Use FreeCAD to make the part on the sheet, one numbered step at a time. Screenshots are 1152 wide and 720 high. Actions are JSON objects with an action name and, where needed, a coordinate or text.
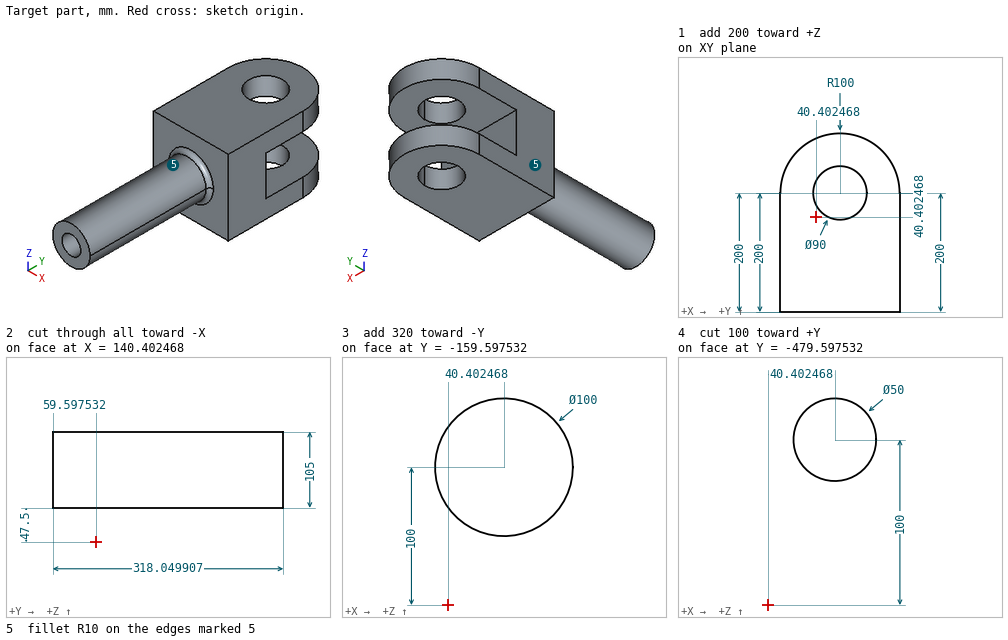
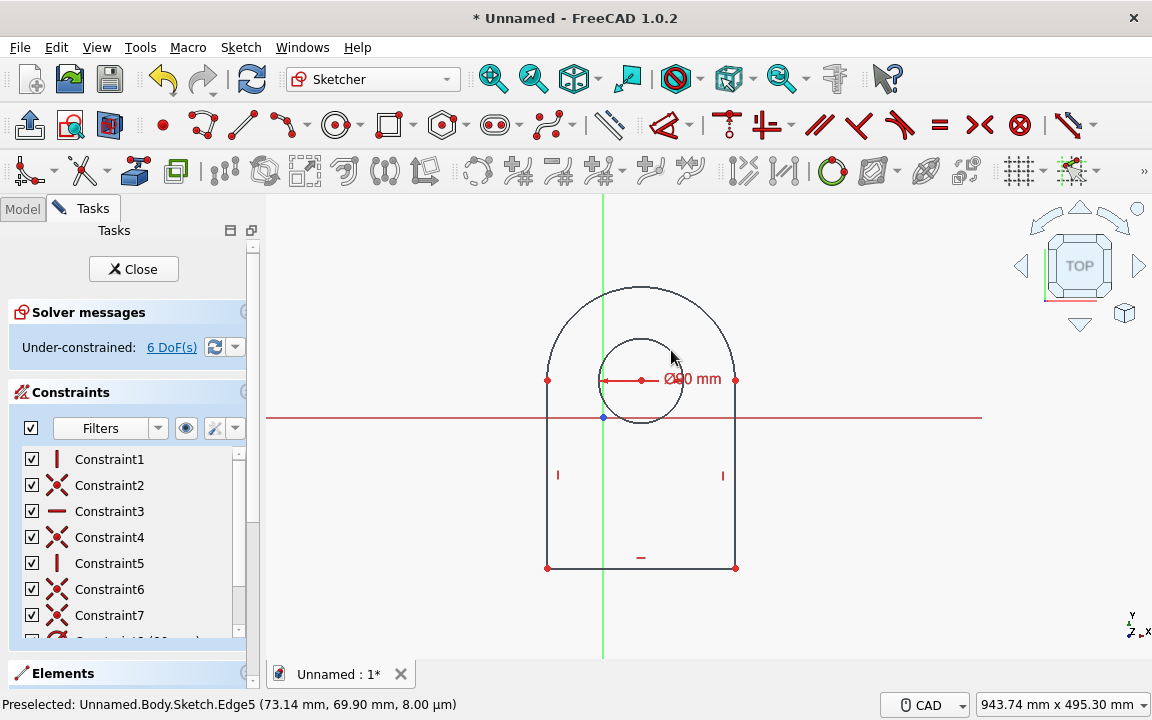
{"action": "left_click", "coordinate": [696, 305]}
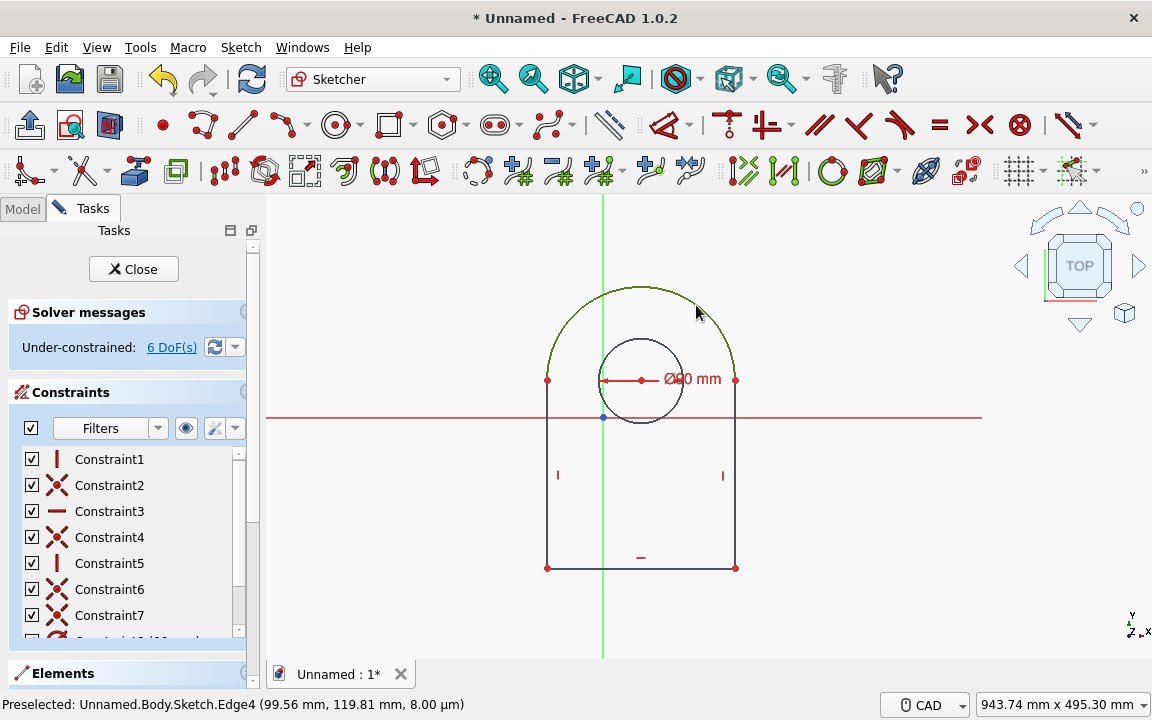
{"action": "key", "text": "k r"}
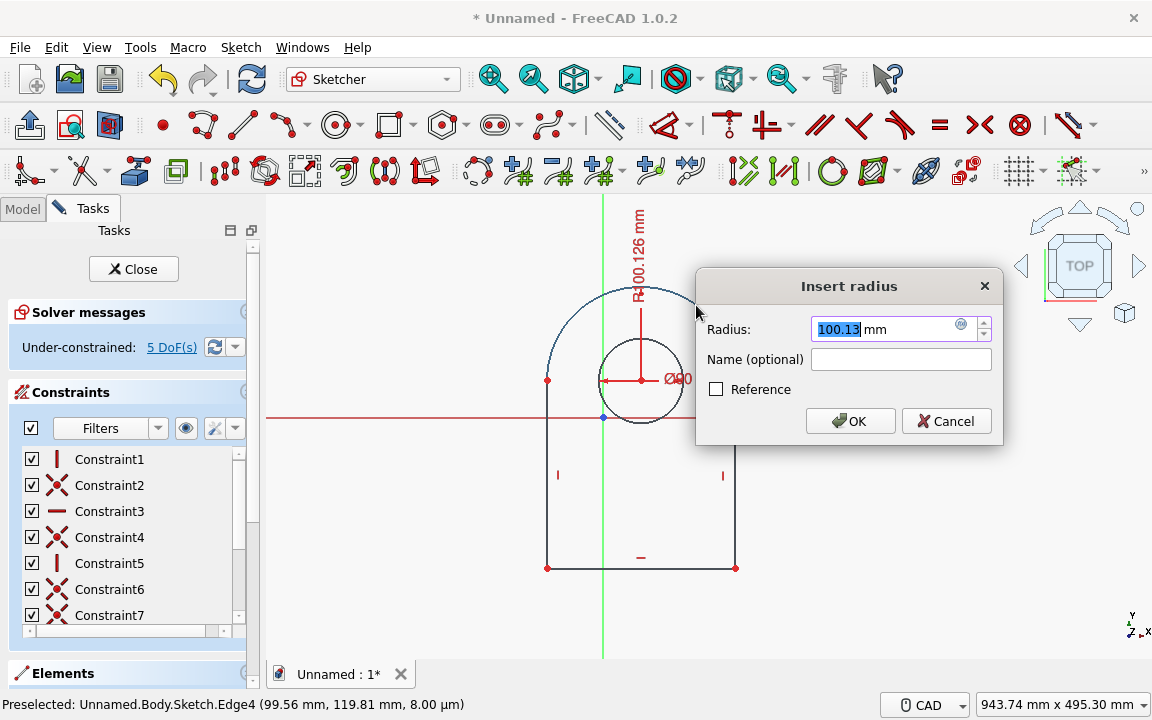
{"action": "type", "text": "100"}
{"action": "key", "text": "Return"}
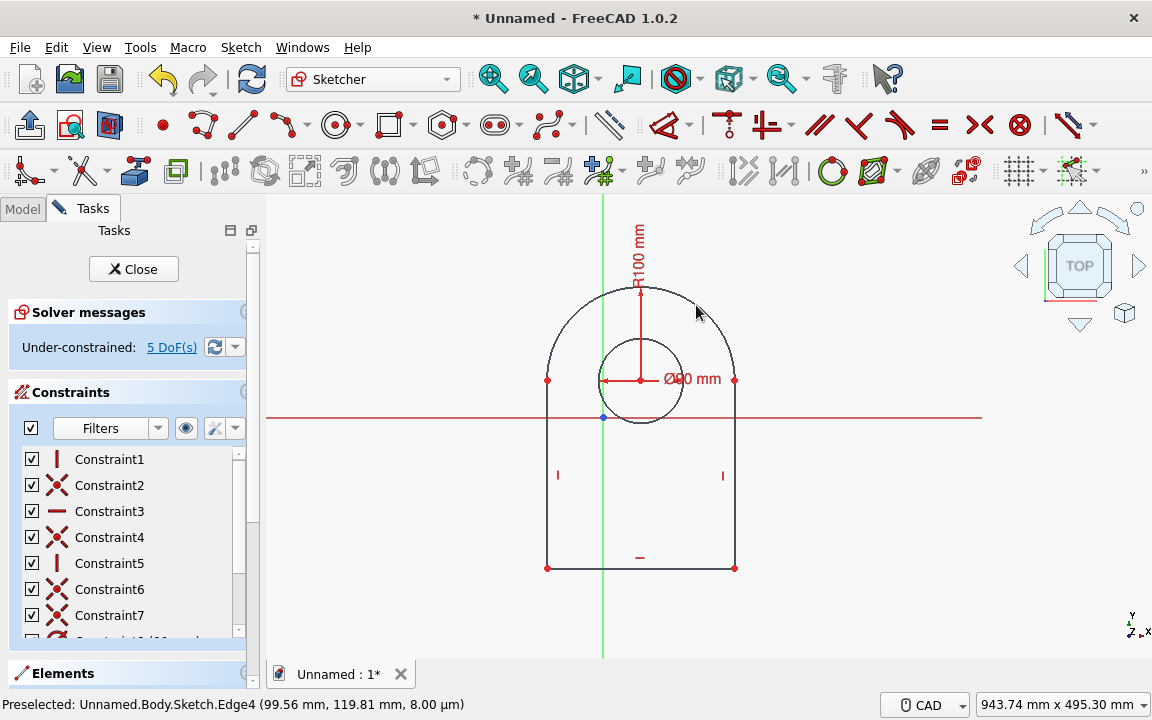
{"action": "left_click", "coordinate": [547, 437]}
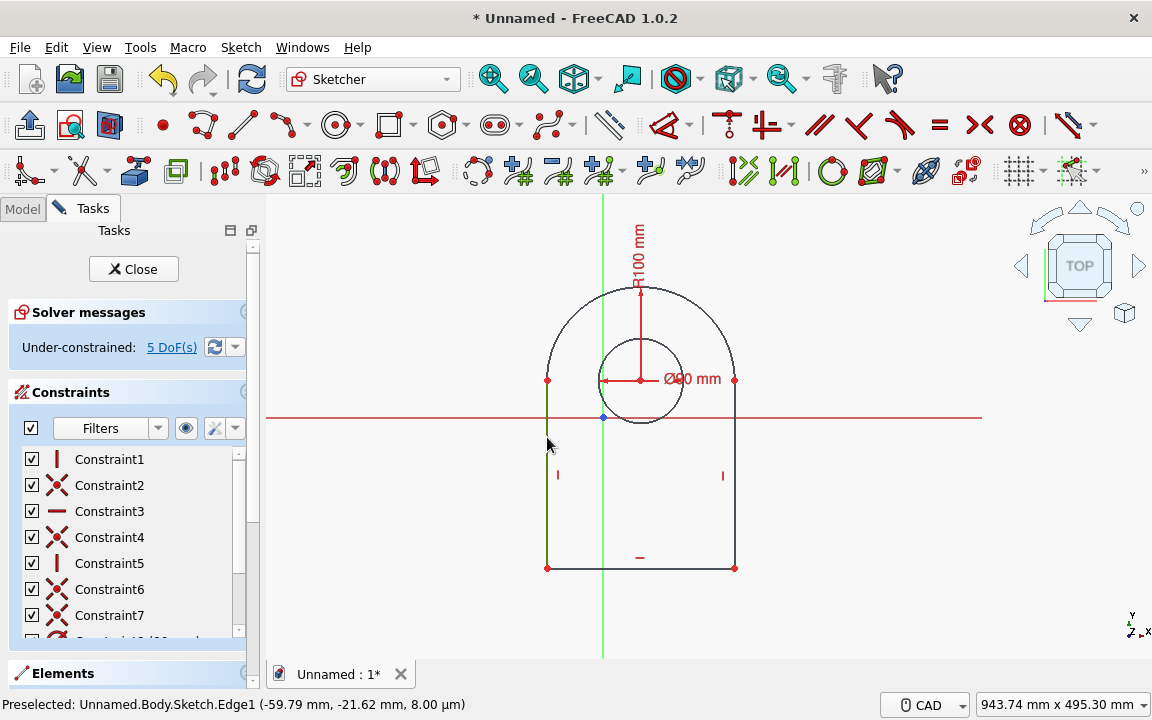
{"action": "key", "text": "i"}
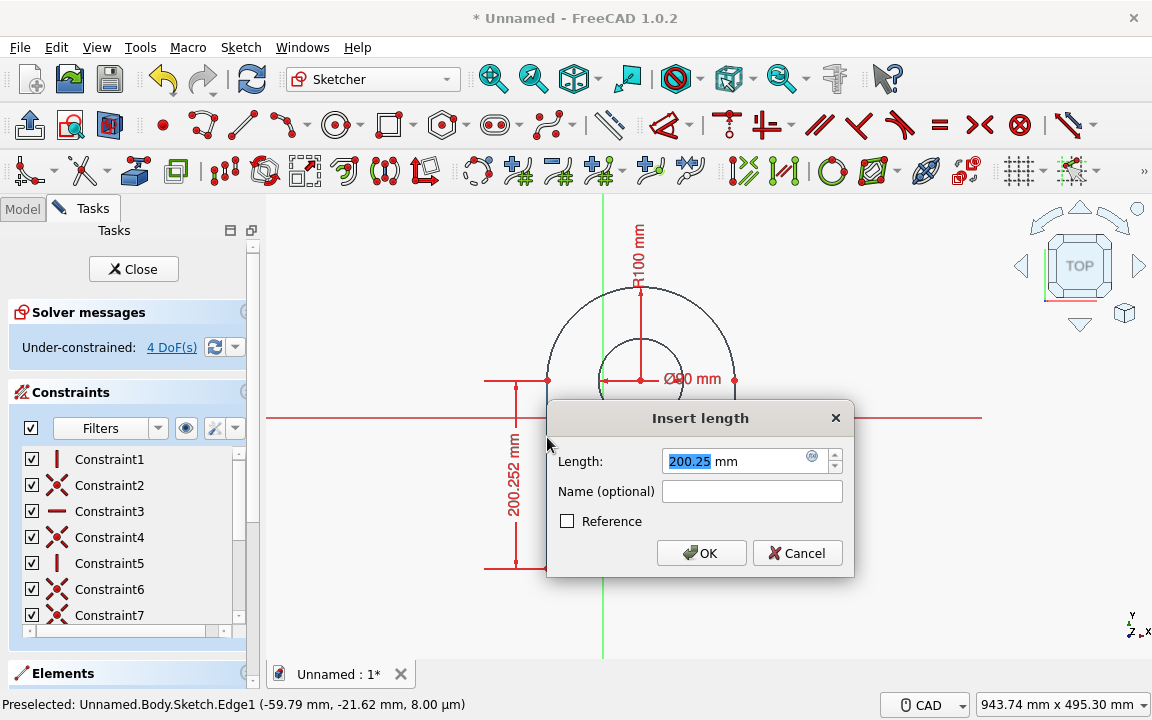
{"action": "type", "text": "200"}
{"action": "key", "text": "Return"}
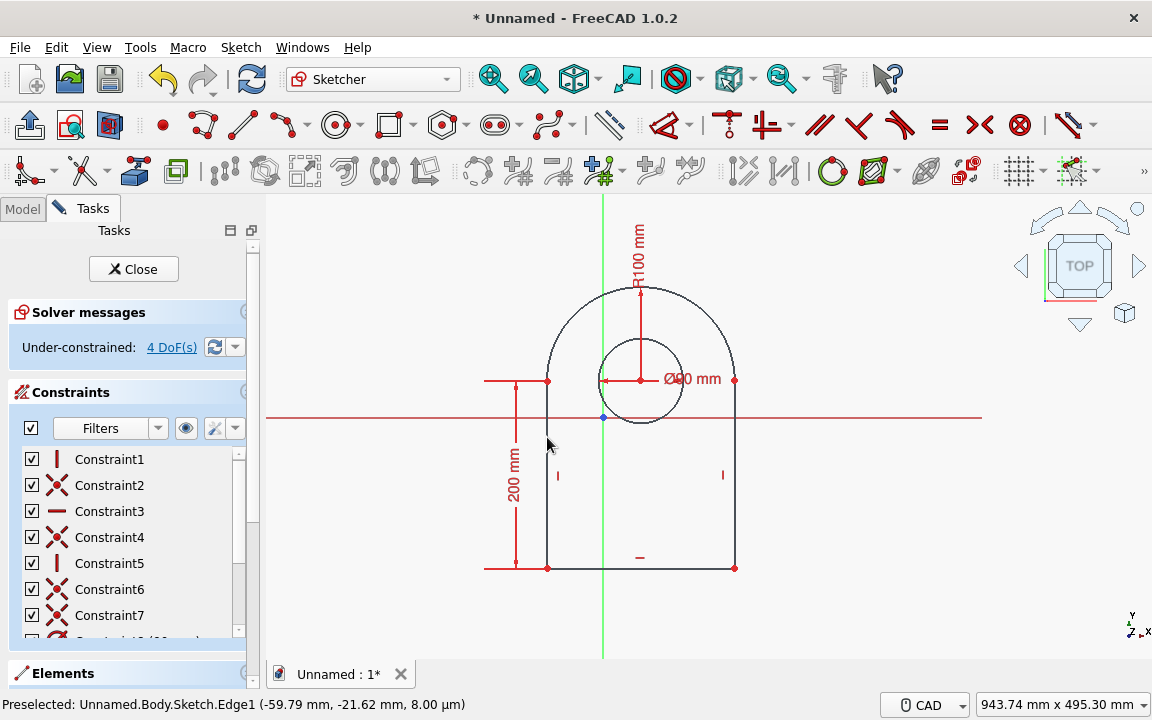
{"action": "left_click", "coordinate": [735, 513]}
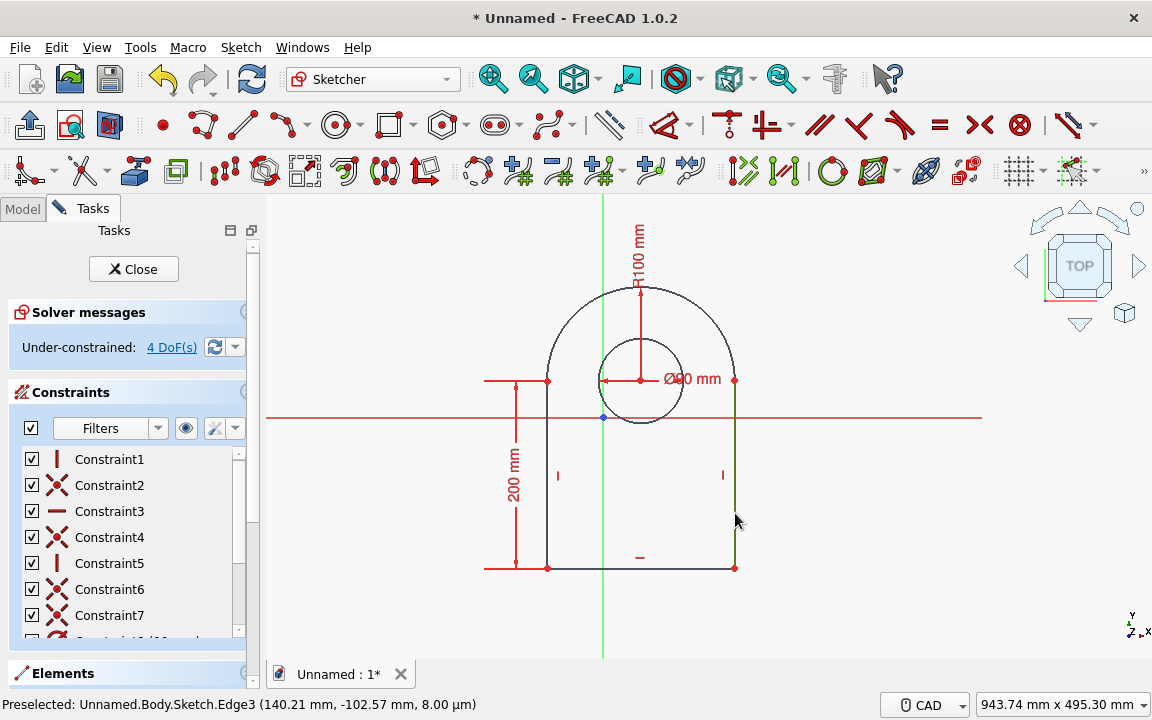
{"action": "key", "text": "i"}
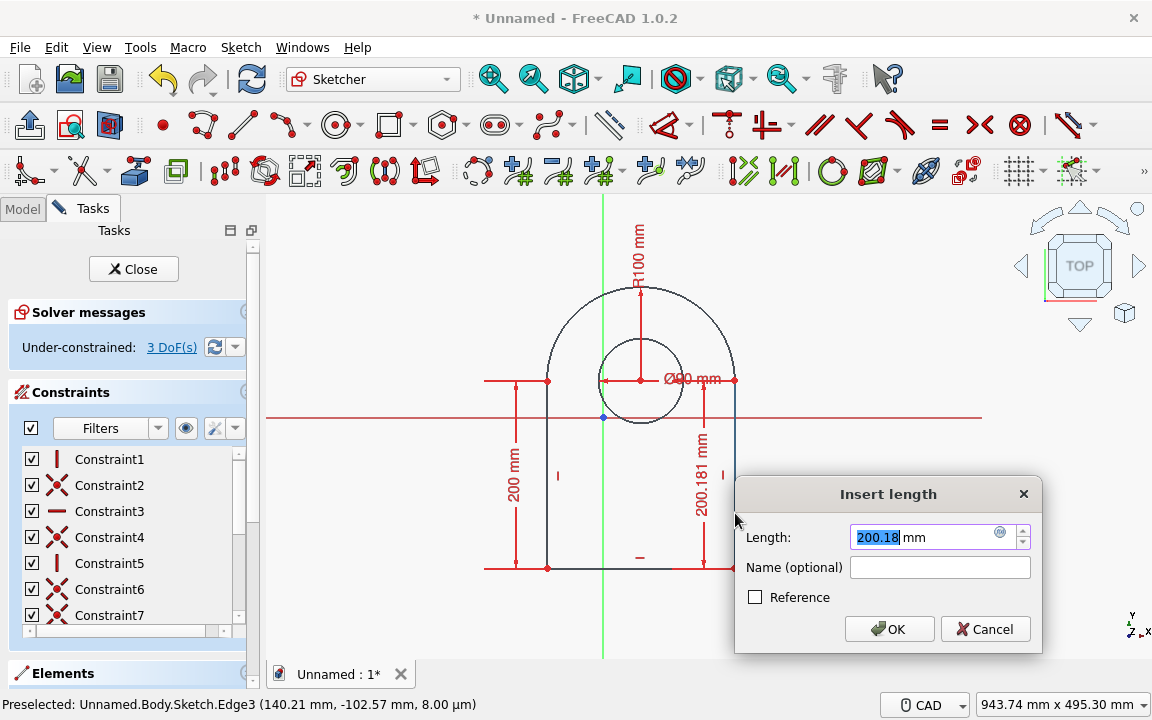
{"action": "type", "text": "200"}
{"action": "key", "text": "Return"}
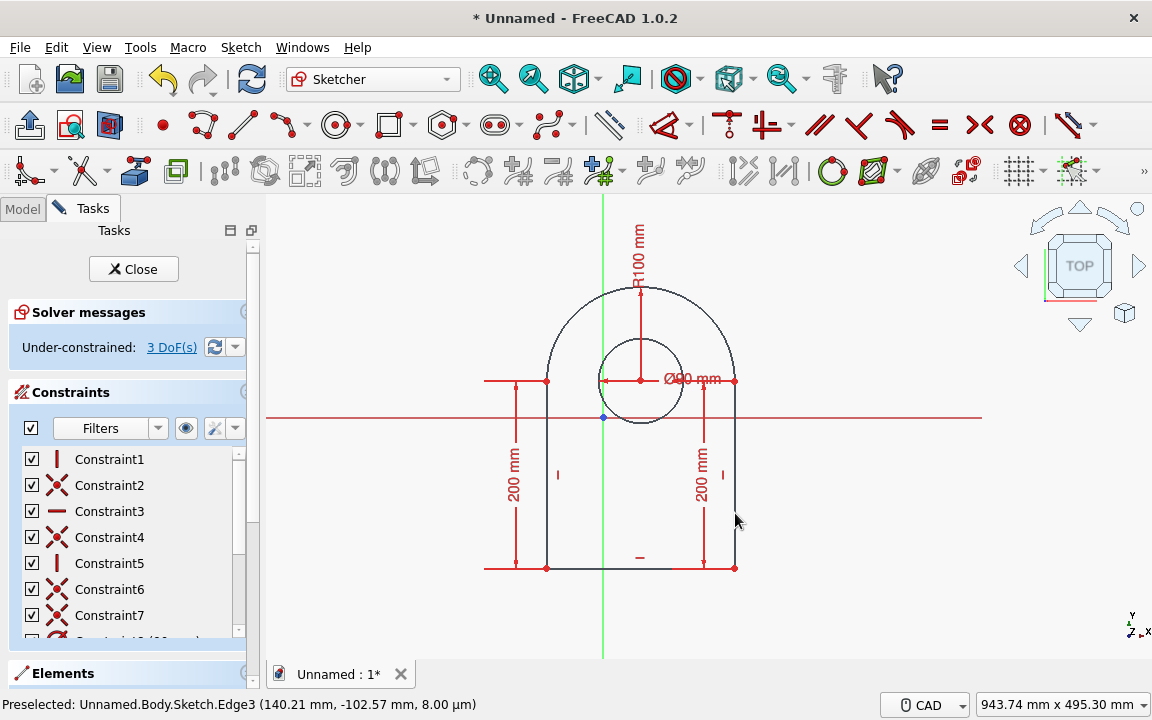
{"action": "left_click", "coordinate": [547, 569]}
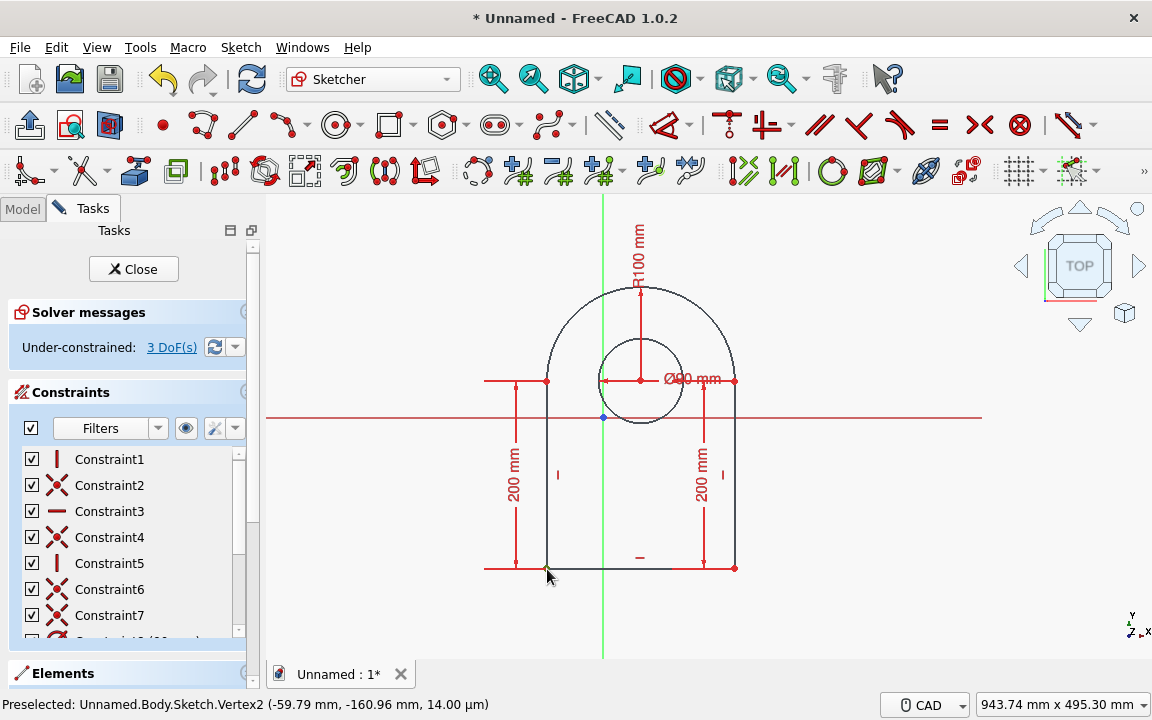
{"action": "left_click", "coordinate": [641, 381]}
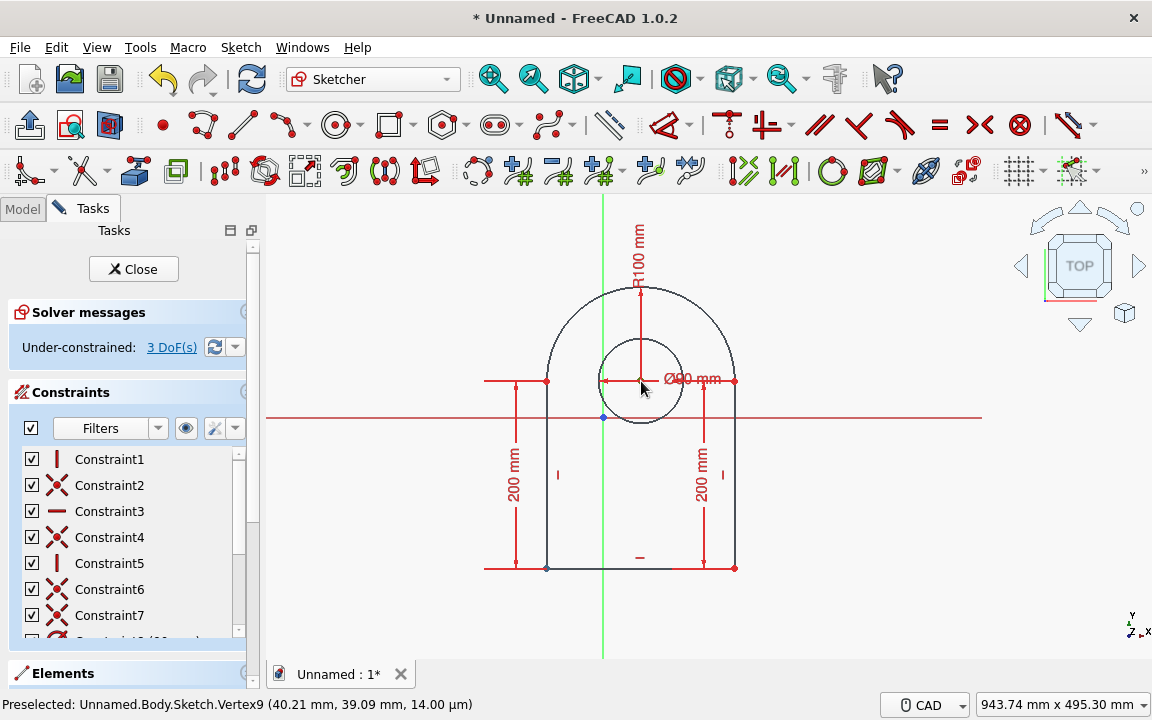
{"action": "left_click", "coordinate": [692, 126]}